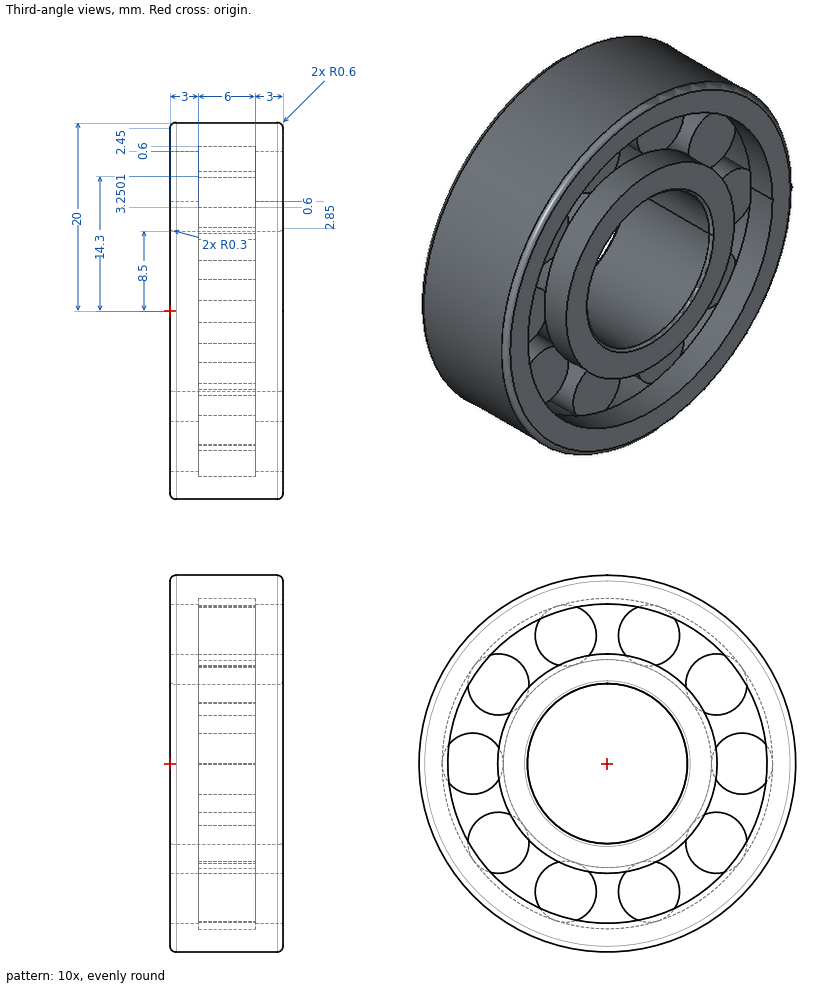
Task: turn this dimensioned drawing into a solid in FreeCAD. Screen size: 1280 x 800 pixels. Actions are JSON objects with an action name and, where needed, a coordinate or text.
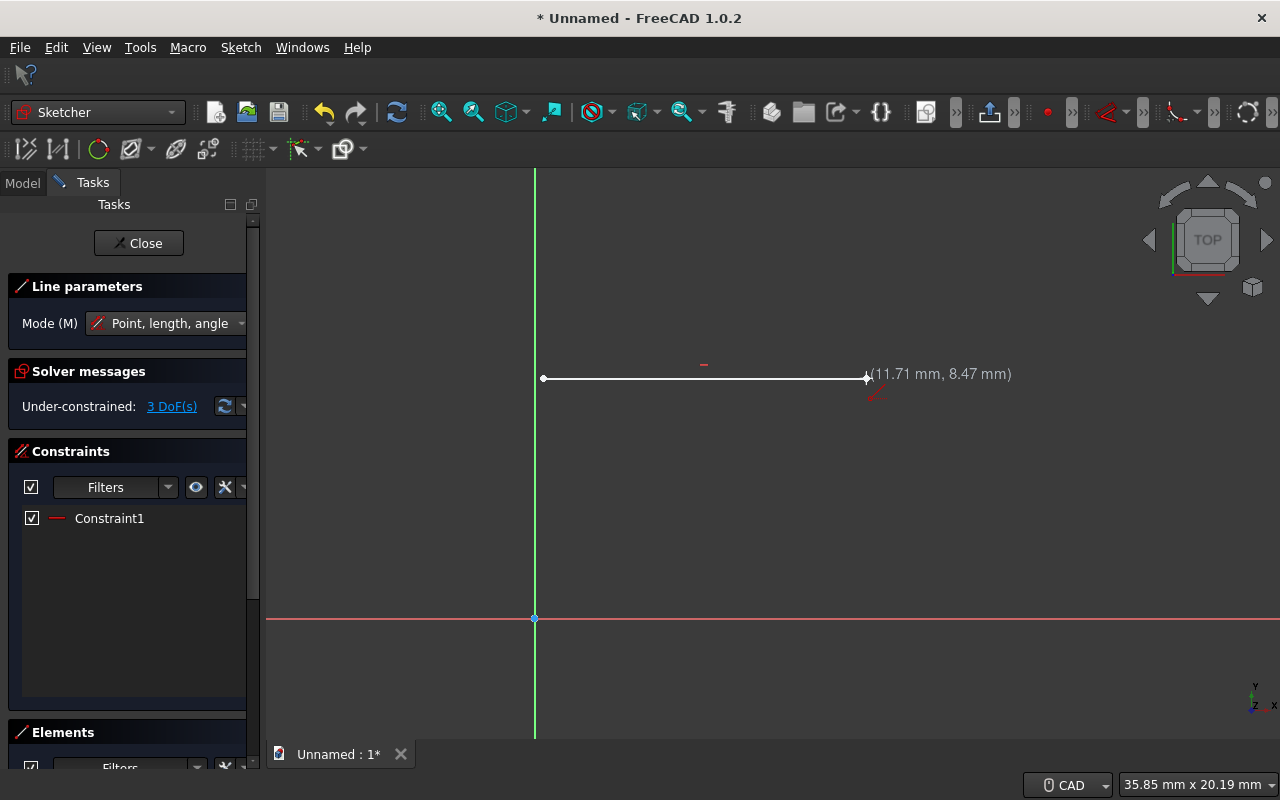
{"action": "key", "text": "g m"}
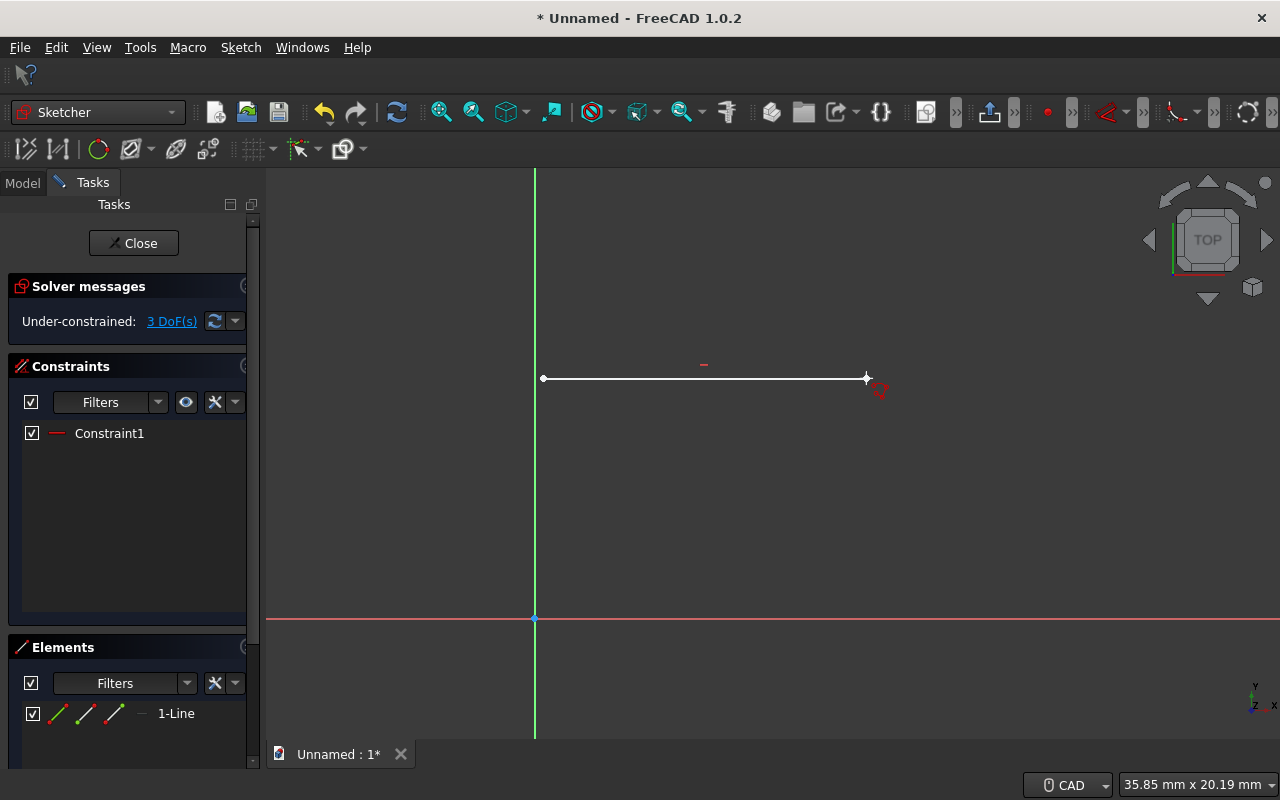
{"action": "scroll", "coordinate": [874, 370], "scroll_direction": "up", "scroll_amount": 2}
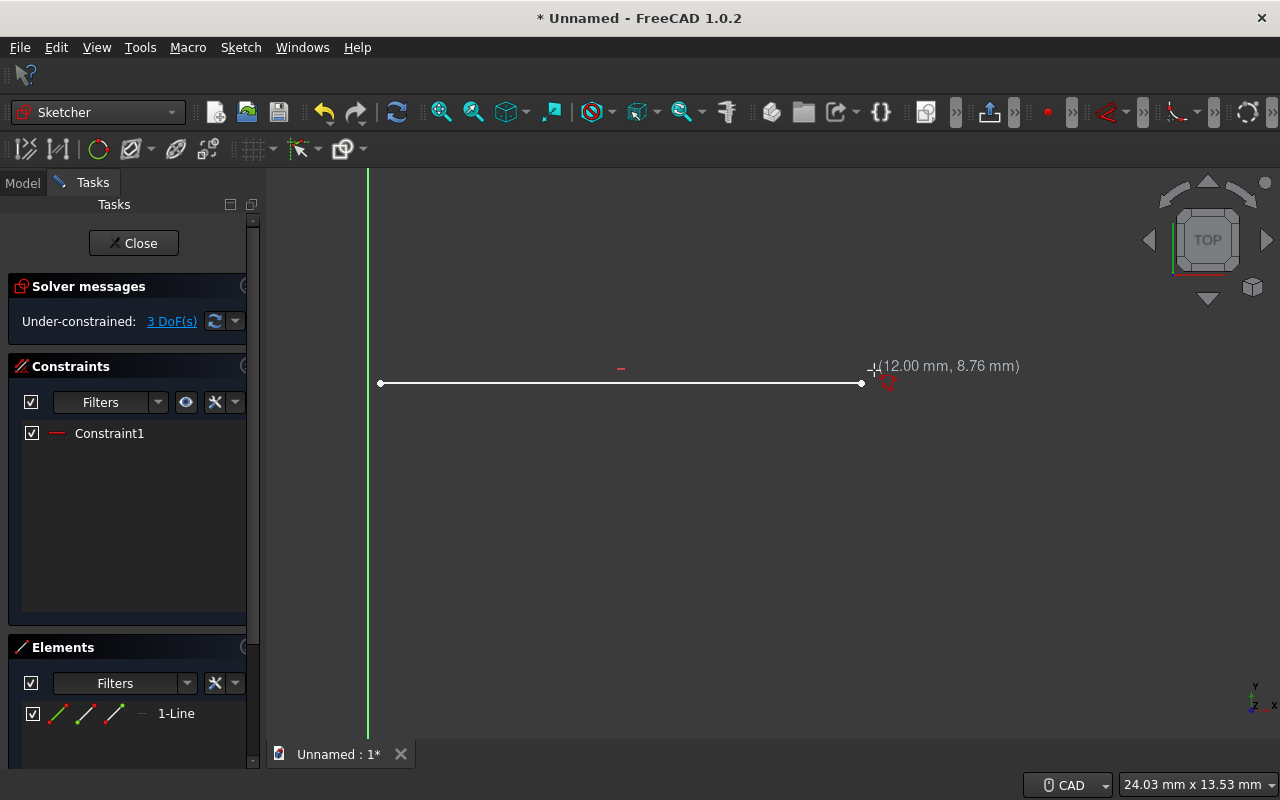
{"action": "left_click", "coordinate": [874, 369]}
{"action": "left_click", "coordinate": [874, 249]}
{"action": "left_click", "coordinate": [747, 249]}
{"action": "left_click", "coordinate": [747, 275]}
{"action": "left_click", "coordinate": [494, 275]}
{"action": "left_click", "coordinate": [494, 249]}
{"action": "left_click", "coordinate": [368, 249]}
{"action": "left_click", "coordinate": [377, 369]}
{"action": "right_click", "coordinate": [377, 369]}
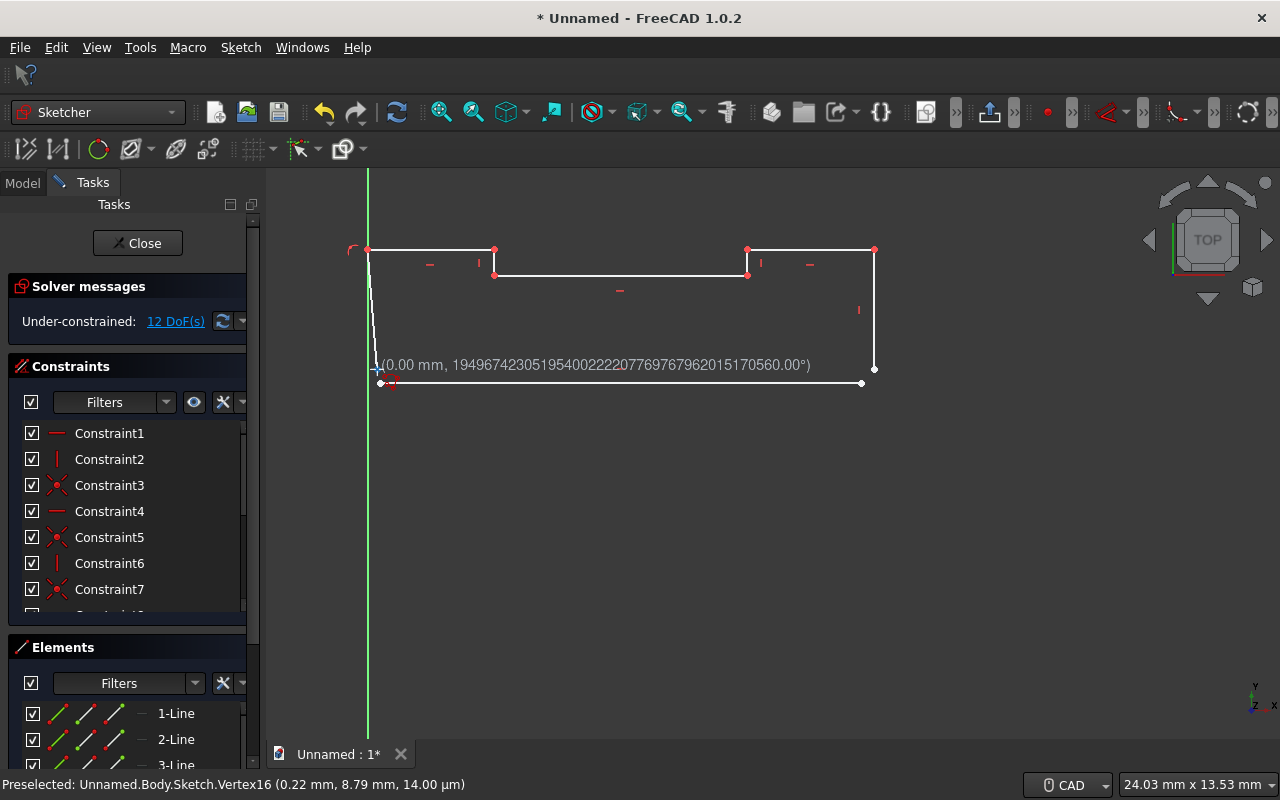
{"action": "key", "text": "g 3 a"}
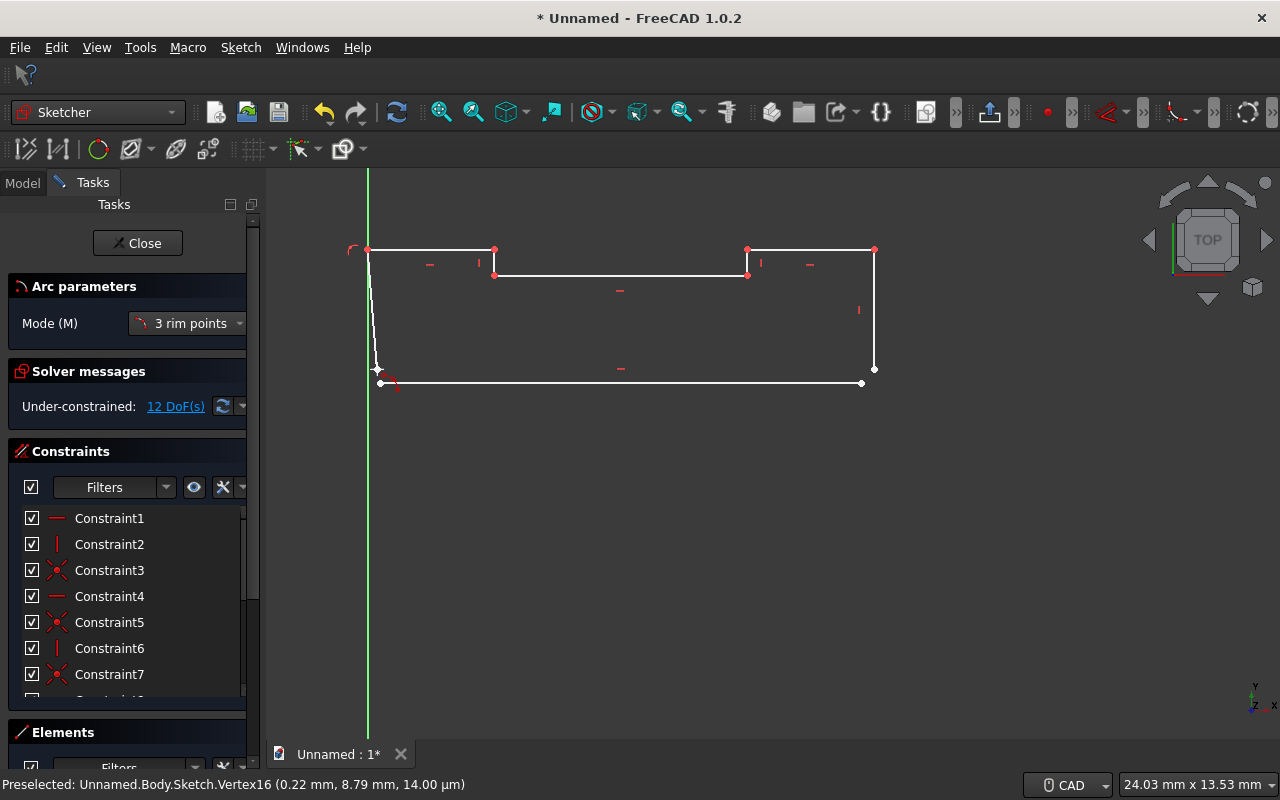
{"action": "left_click", "coordinate": [862, 383]}
{"action": "left_click", "coordinate": [874, 370]}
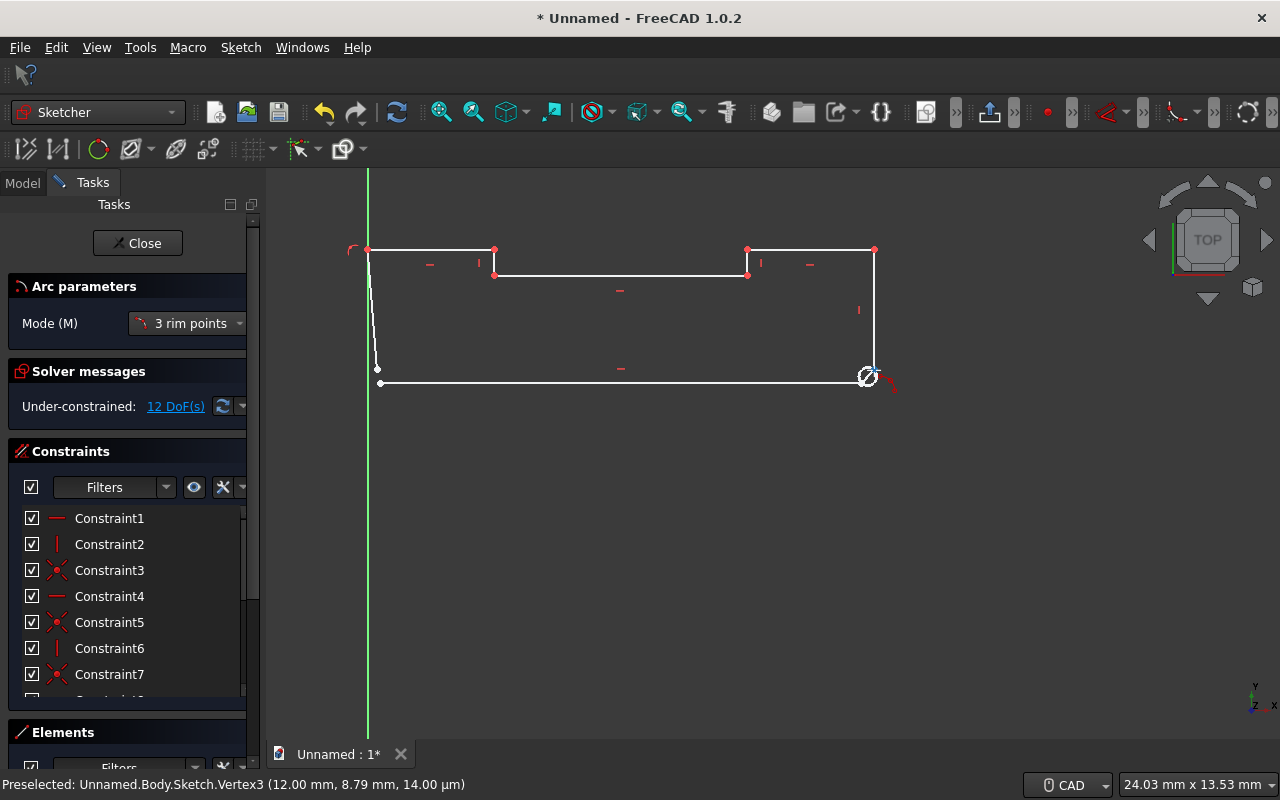
{"action": "scroll", "coordinate": [870, 378], "scroll_direction": "up", "scroll_amount": 8}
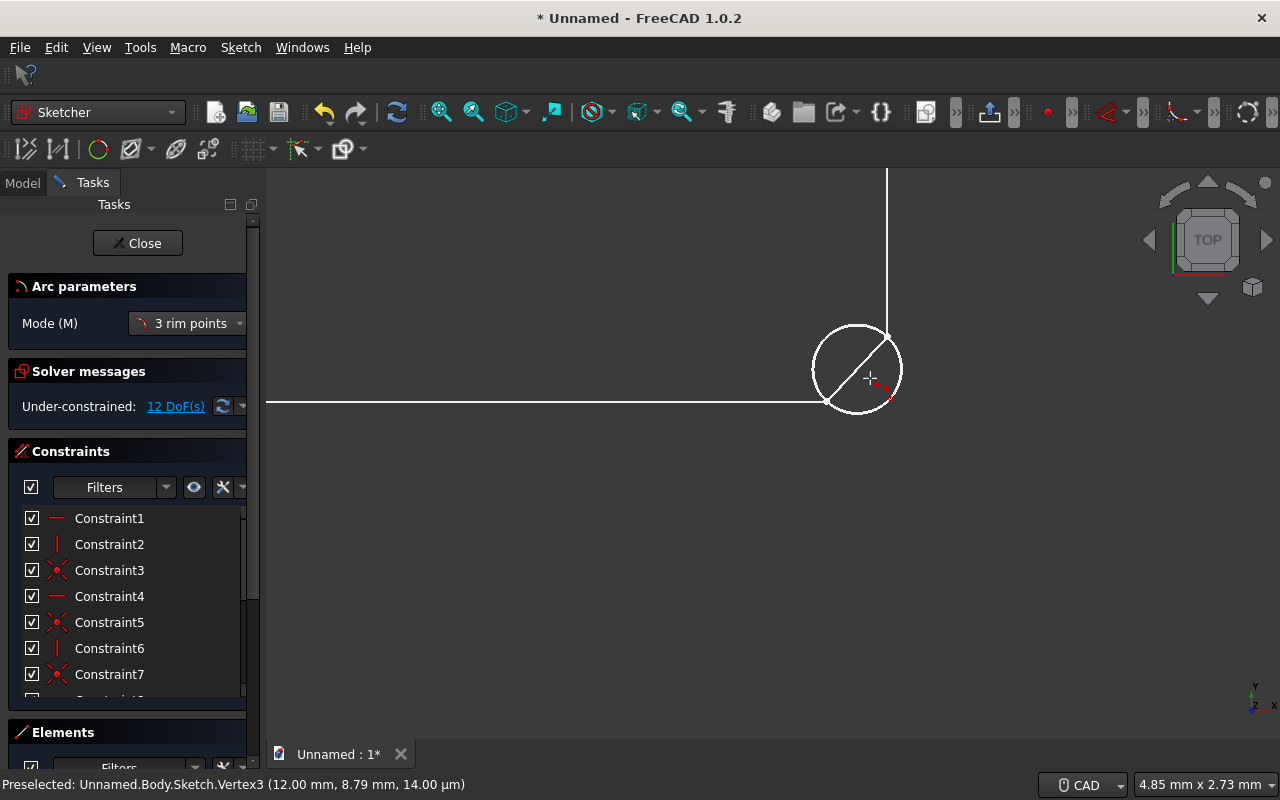
{"action": "left_click", "coordinate": [868, 378]}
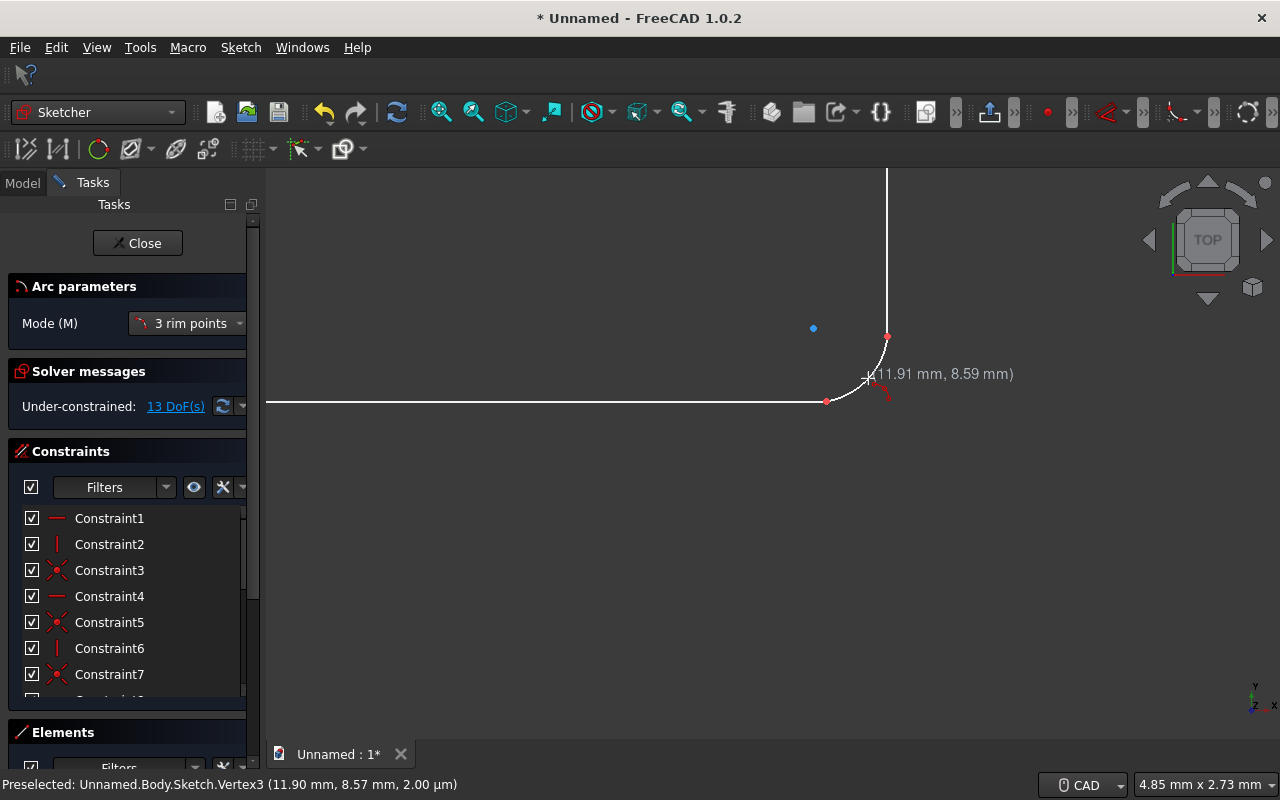
{"action": "scroll", "coordinate": [872, 375], "scroll_direction": "down", "scroll_amount": 10}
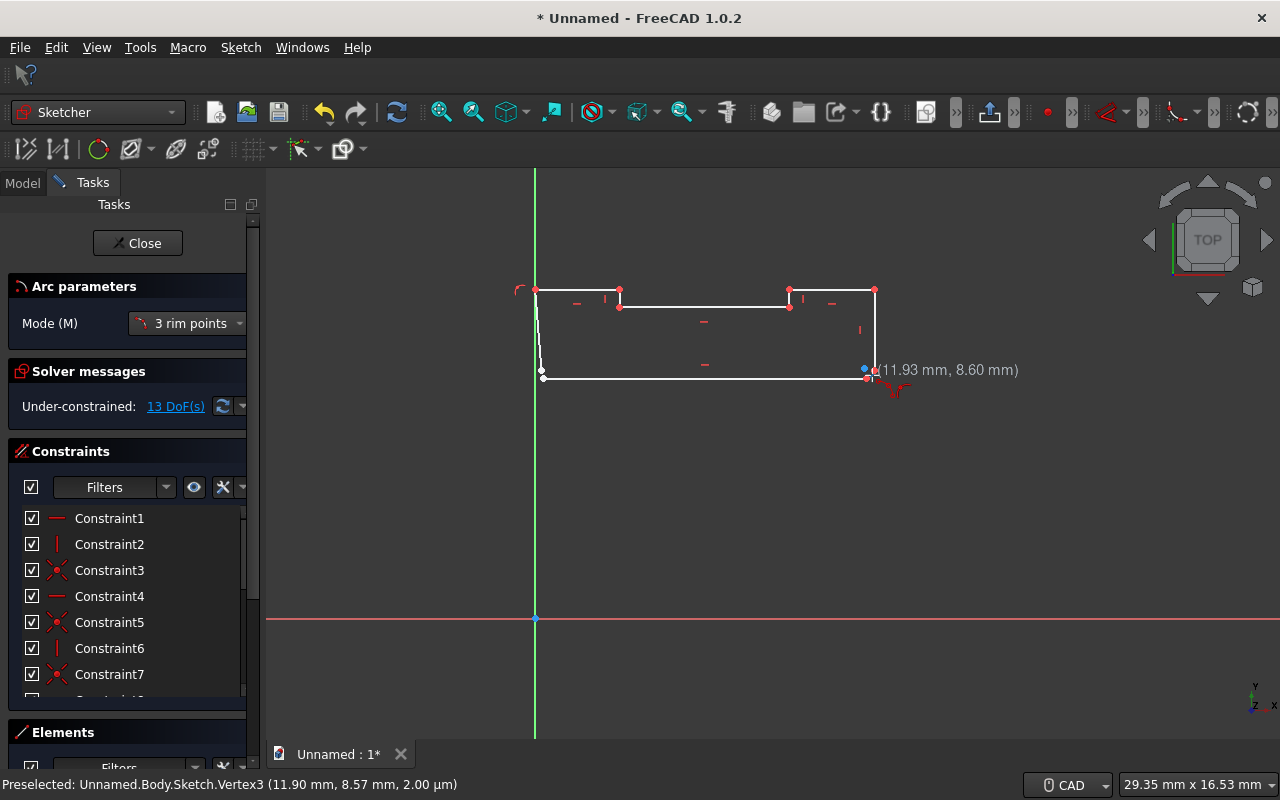
{"action": "scroll", "coordinate": [535, 370], "scroll_direction": "up", "scroll_amount": 2}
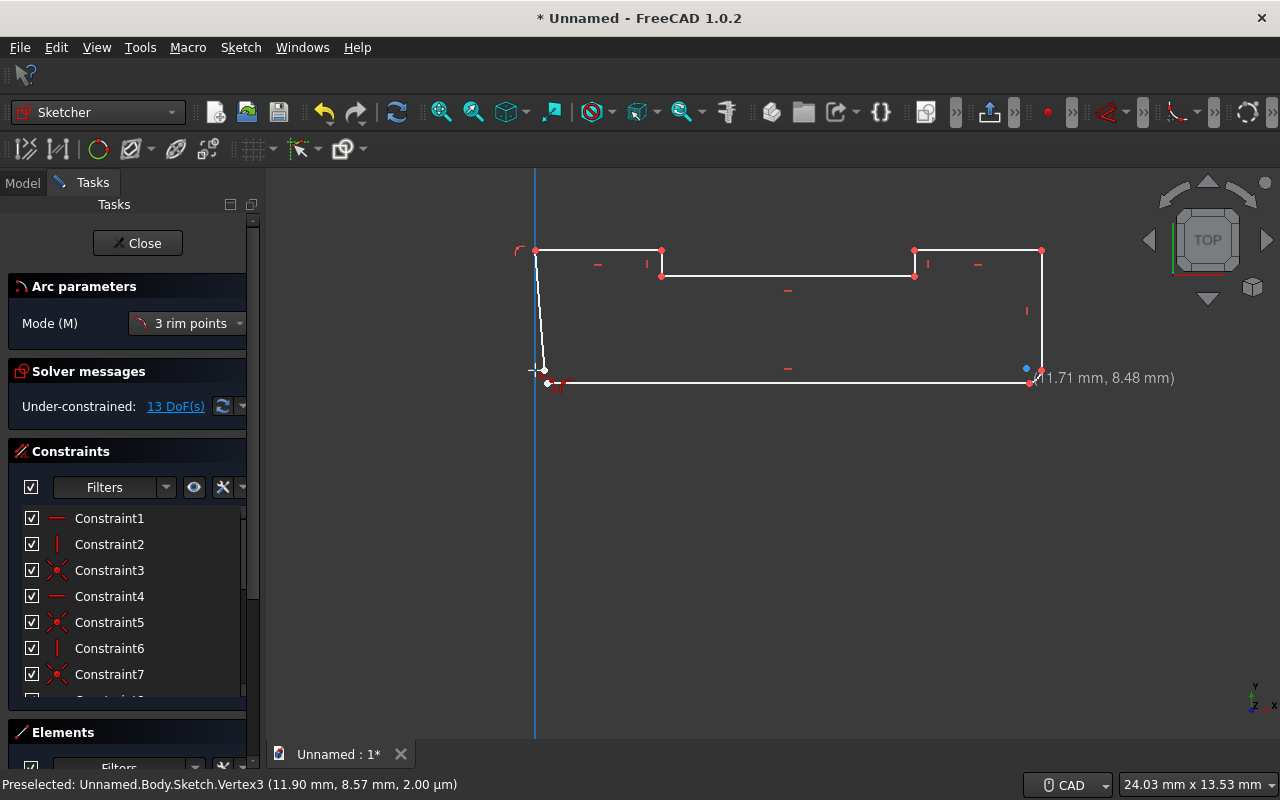
{"action": "left_click", "coordinate": [545, 370]}